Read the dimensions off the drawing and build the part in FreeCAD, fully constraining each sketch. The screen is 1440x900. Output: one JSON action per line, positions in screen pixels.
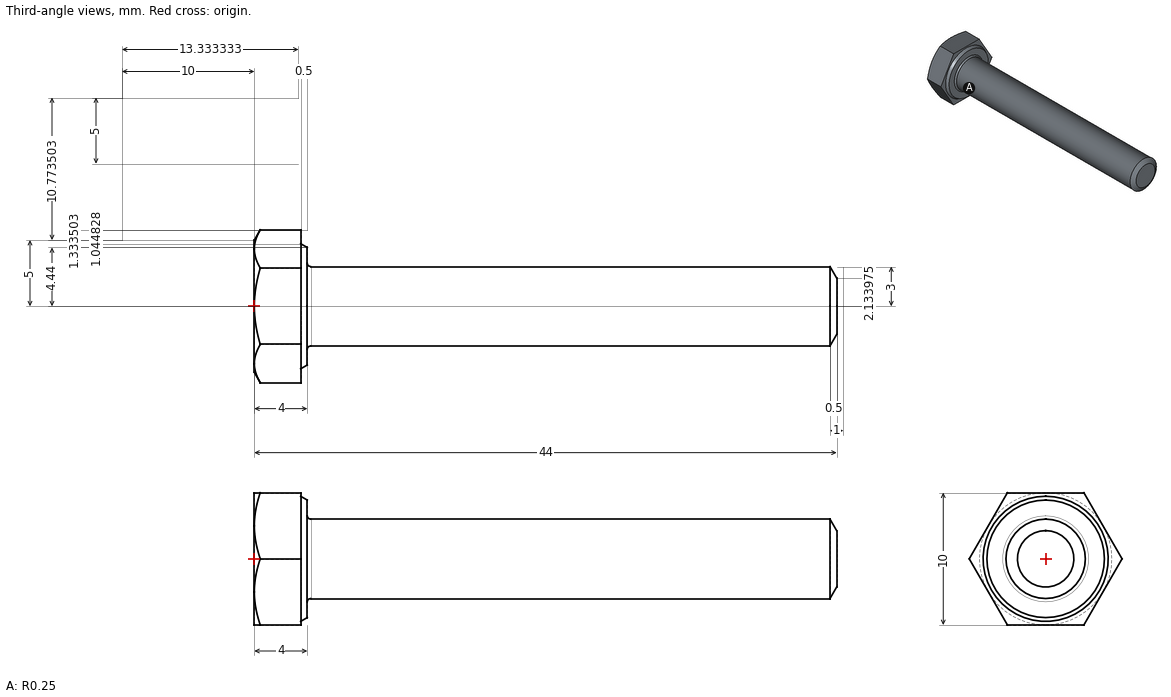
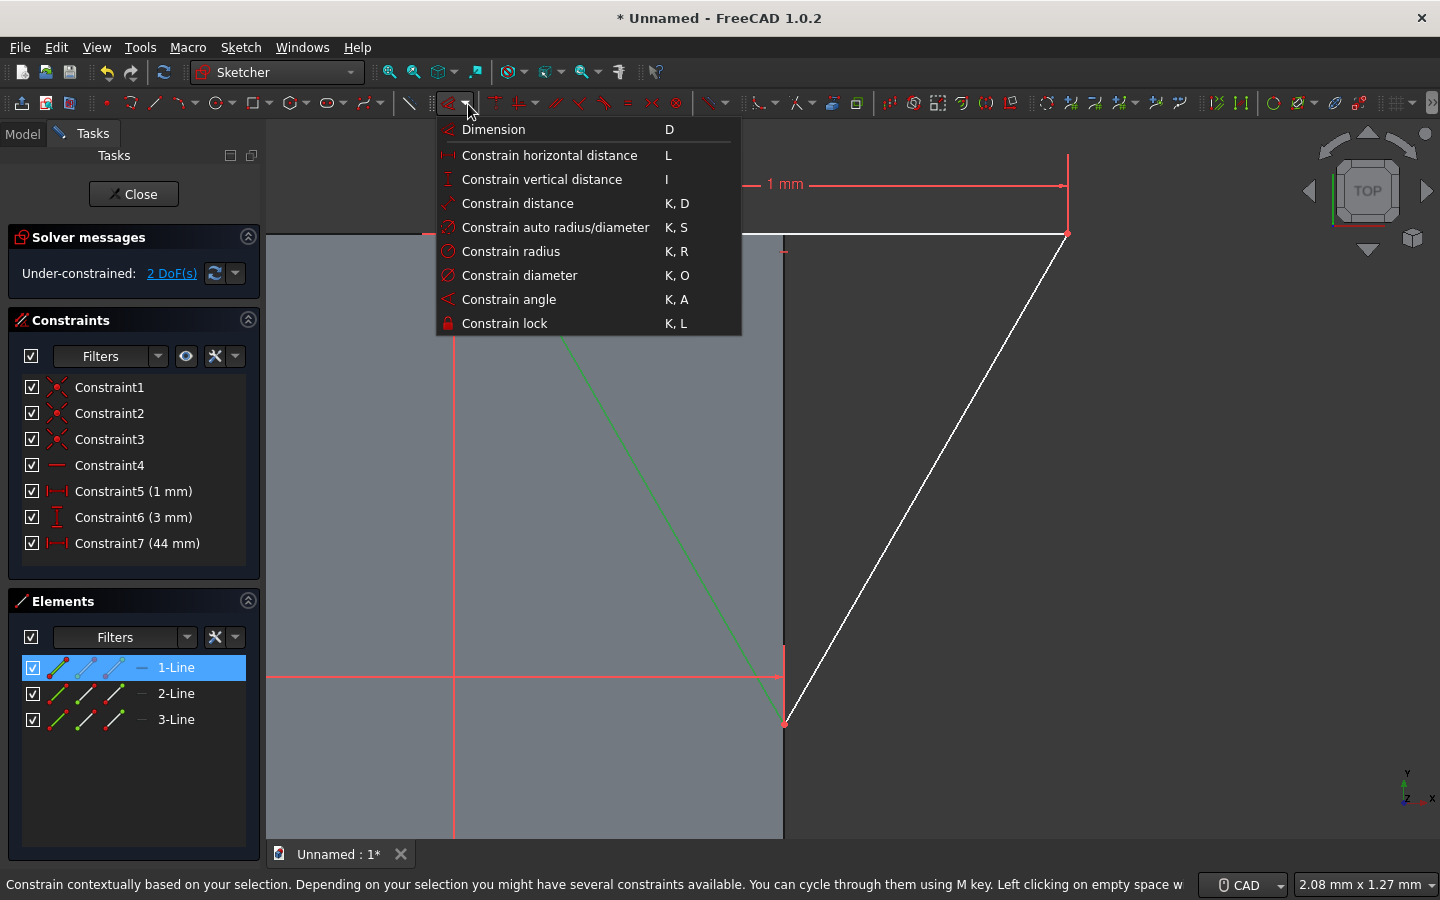
{"action": "left_click", "coordinate": [589, 155]}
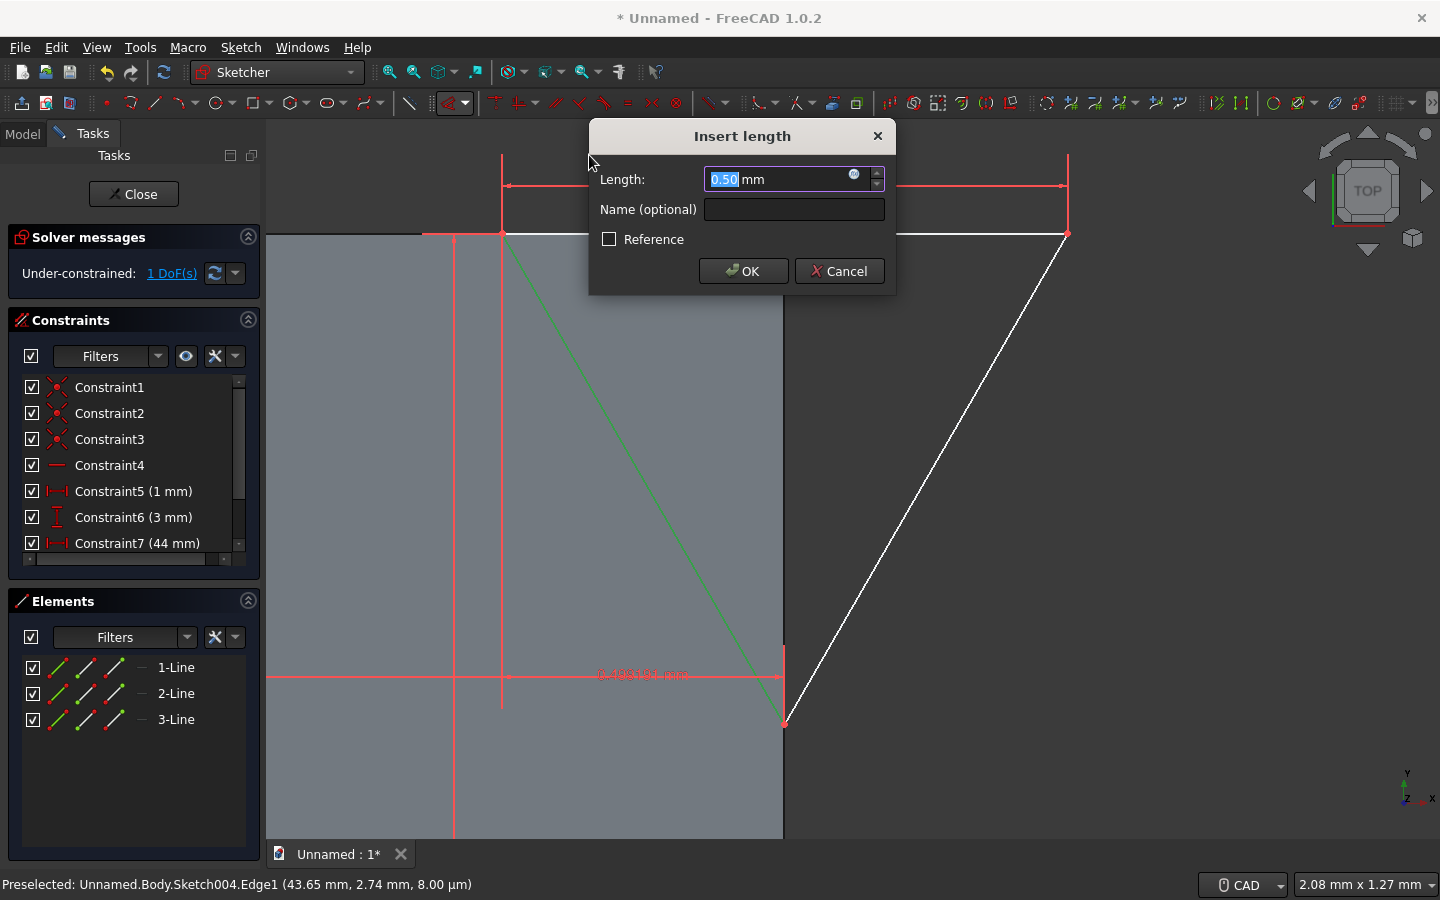
{"action": "type", "text": "0.5"}
{"action": "key", "text": "Return"}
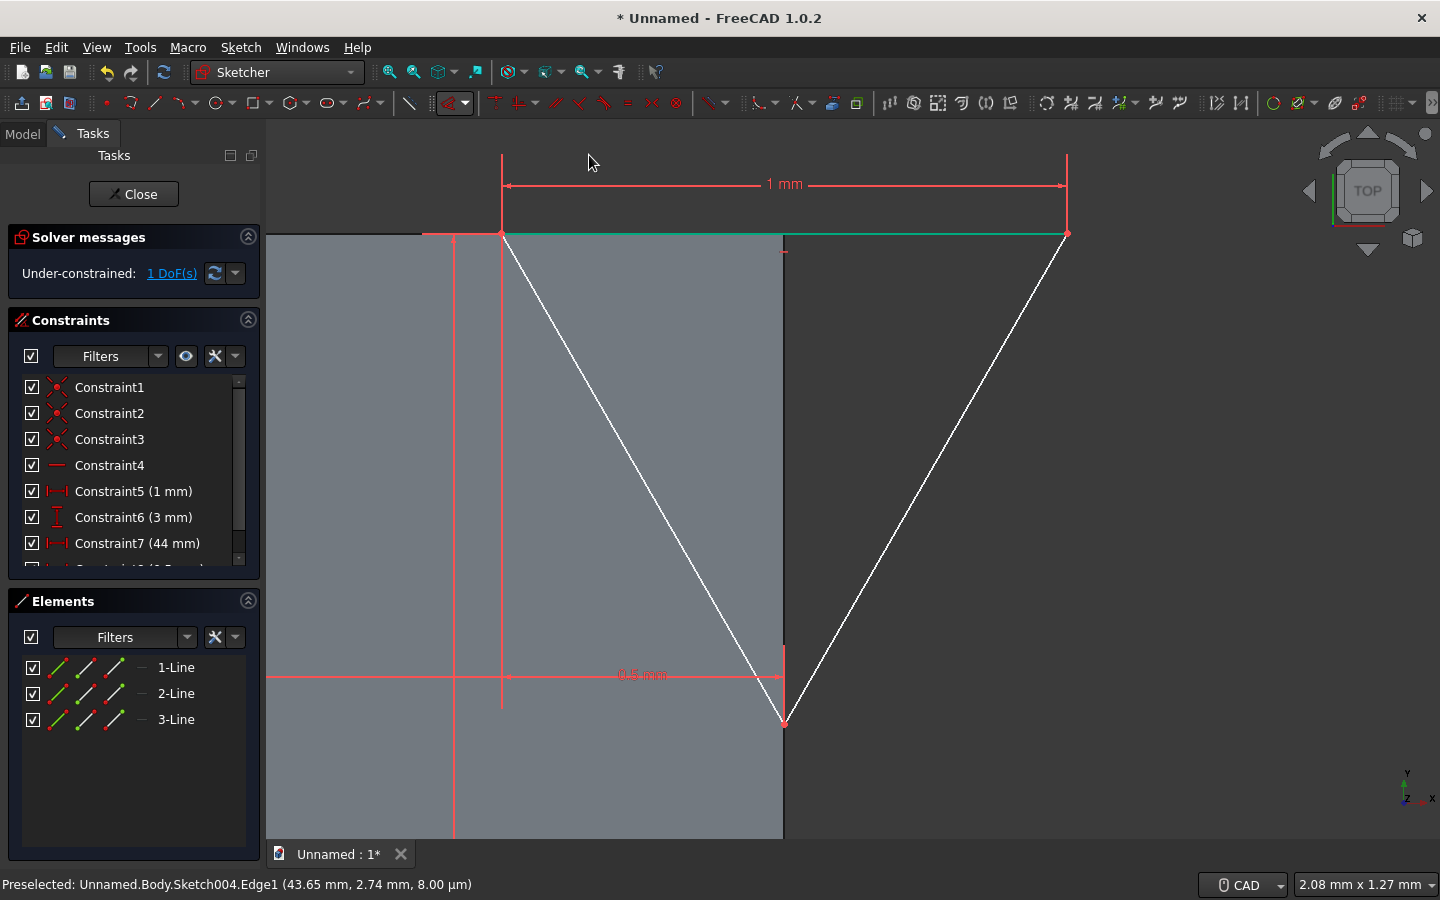
{"action": "left_click", "coordinate": [784, 725]}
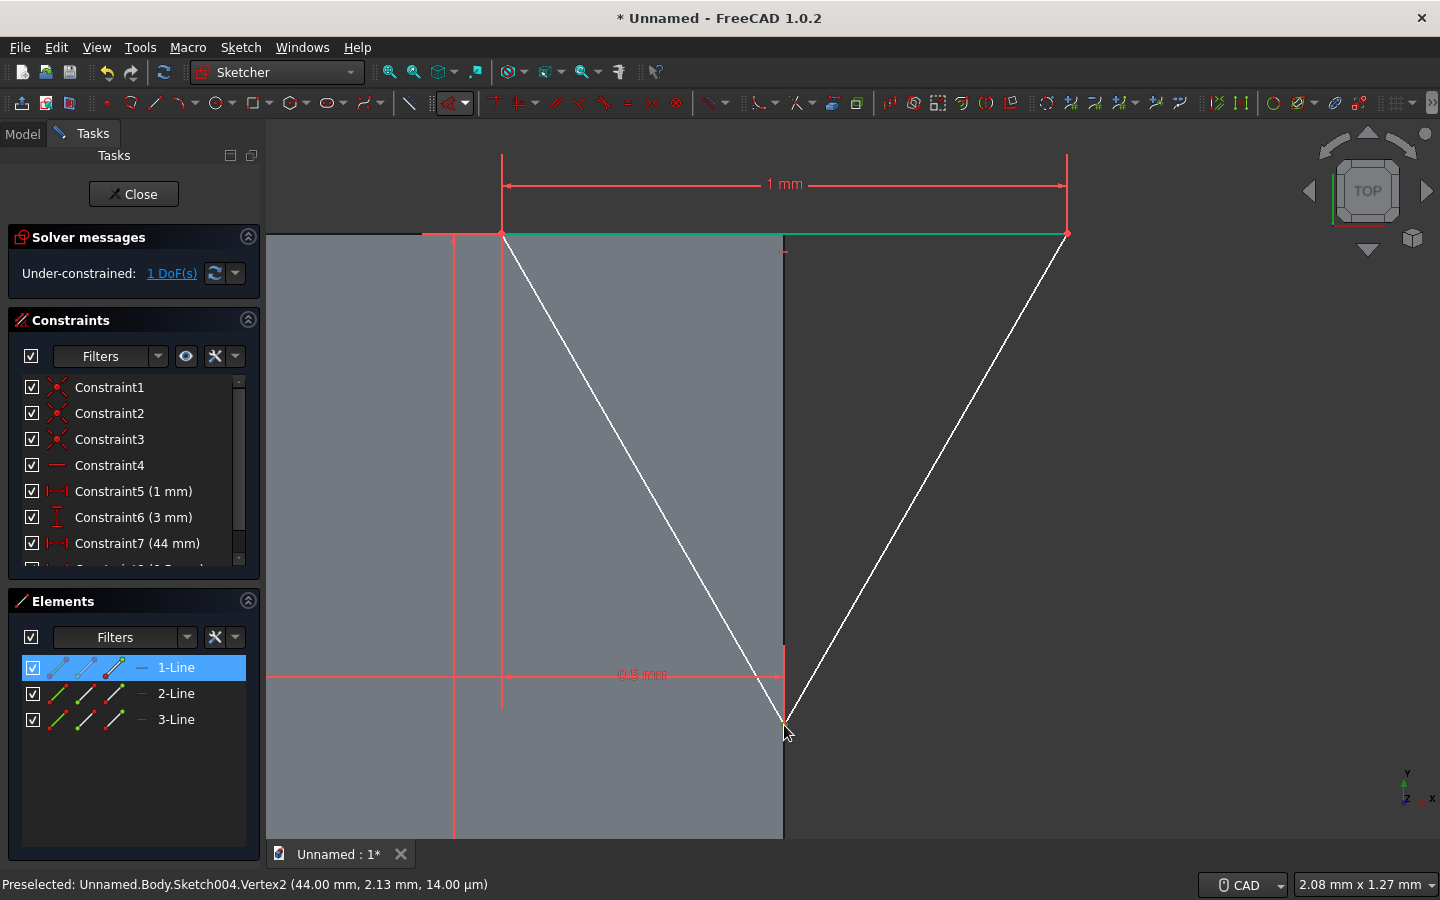
{"action": "left_click", "coordinate": [468, 104]}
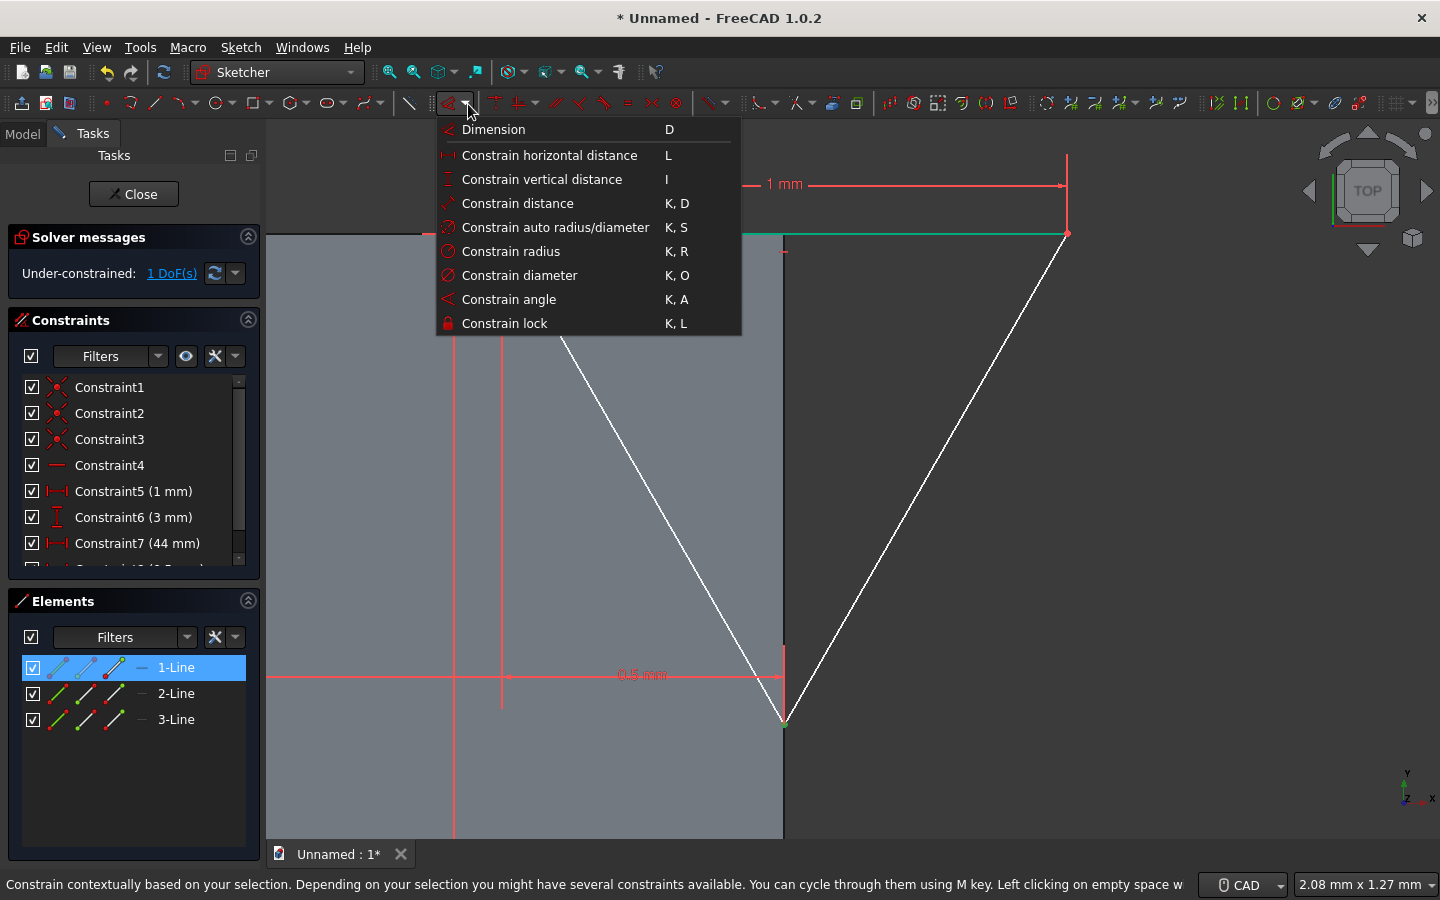
{"action": "left_click", "coordinate": [589, 179]}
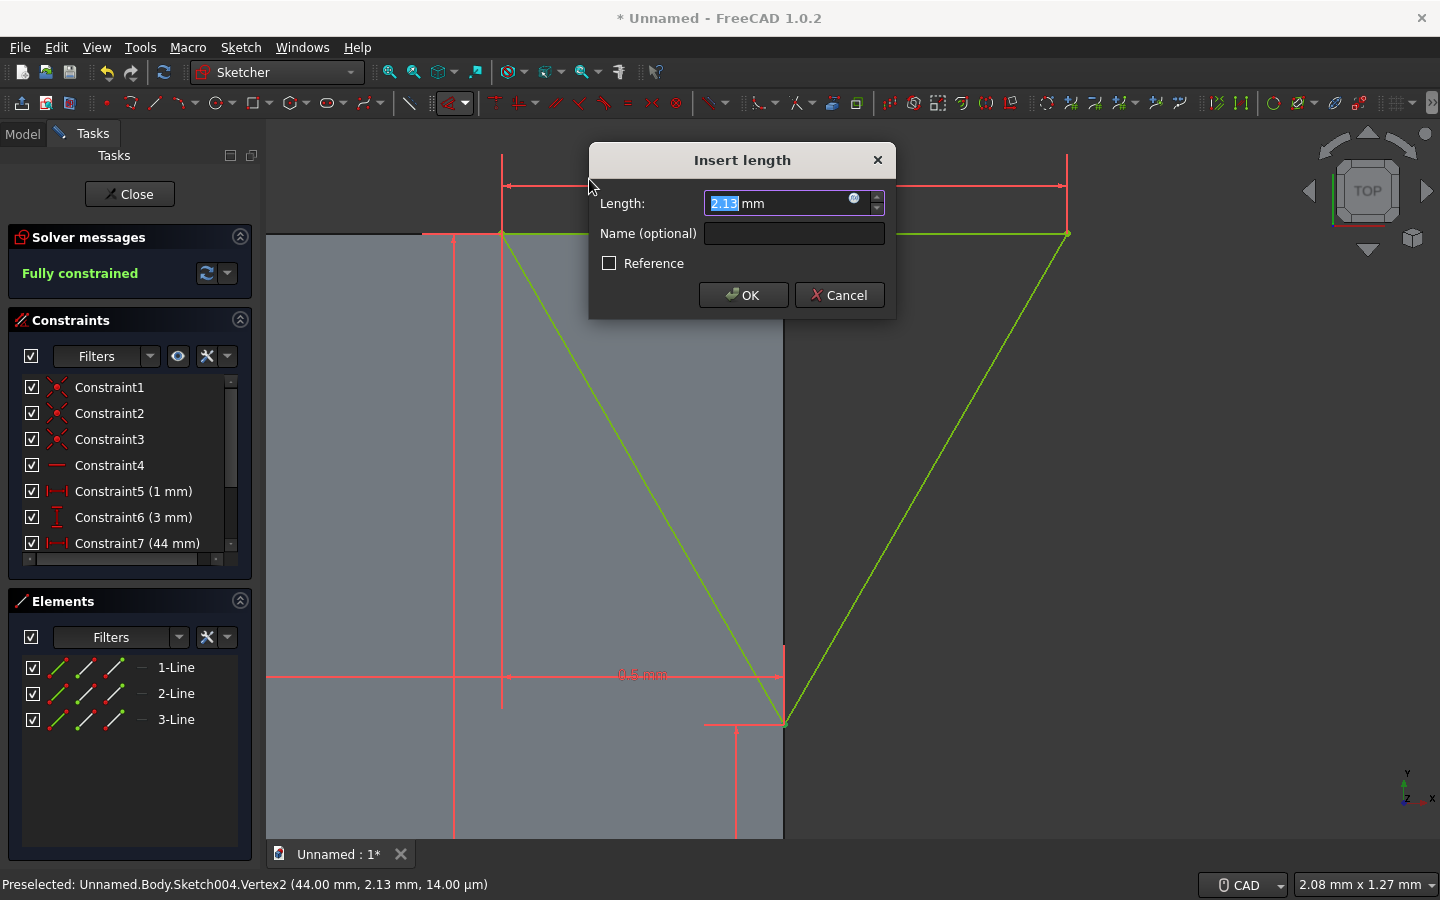
{"action": "type", "text": "2.133975"}
{"action": "key", "text": "Return"}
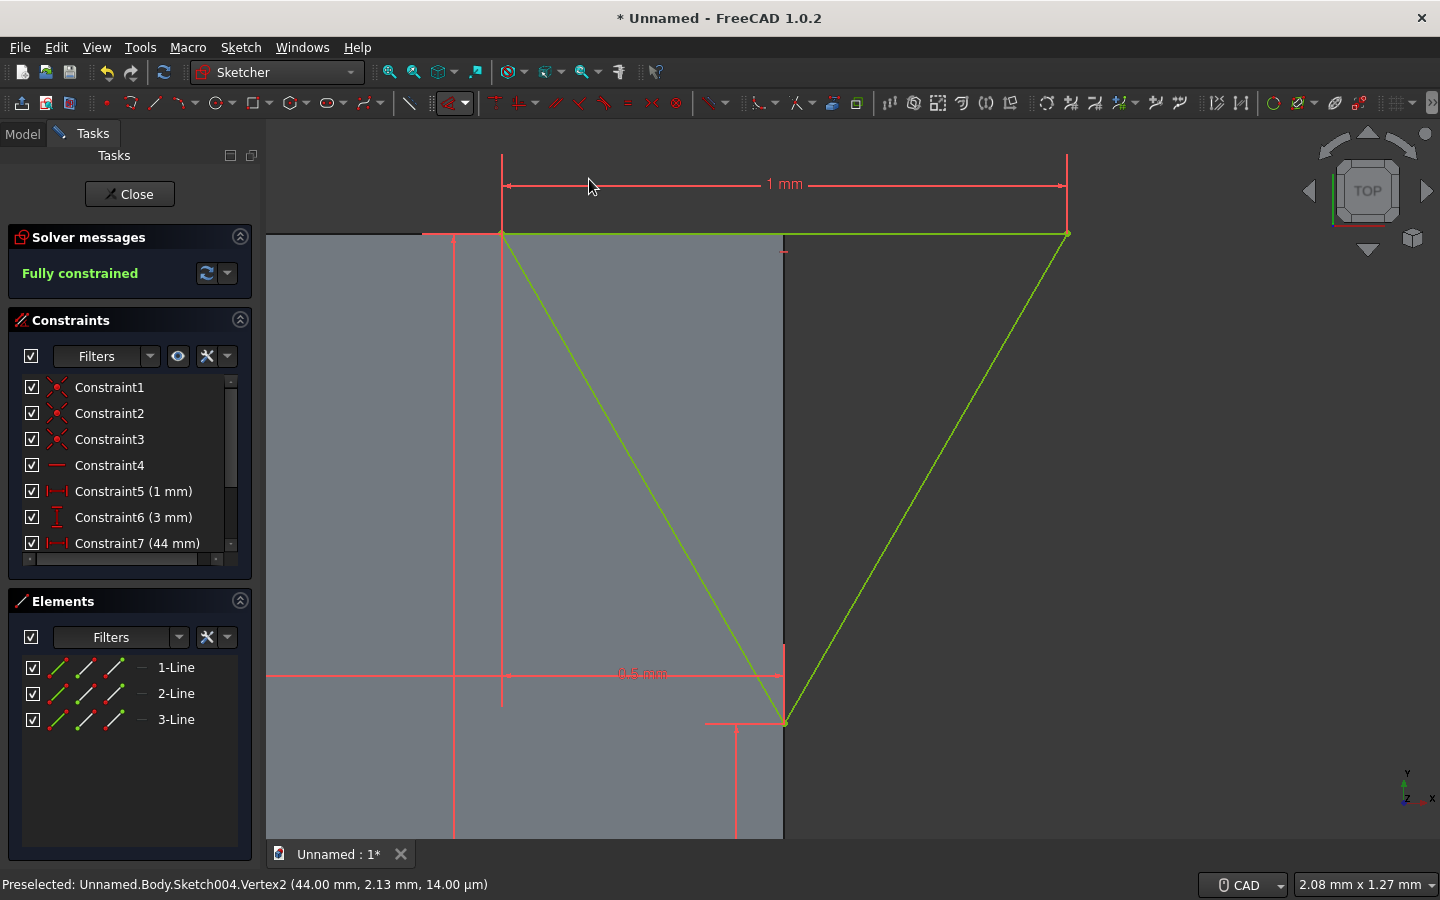
{"action": "left_click", "coordinate": [130, 194]}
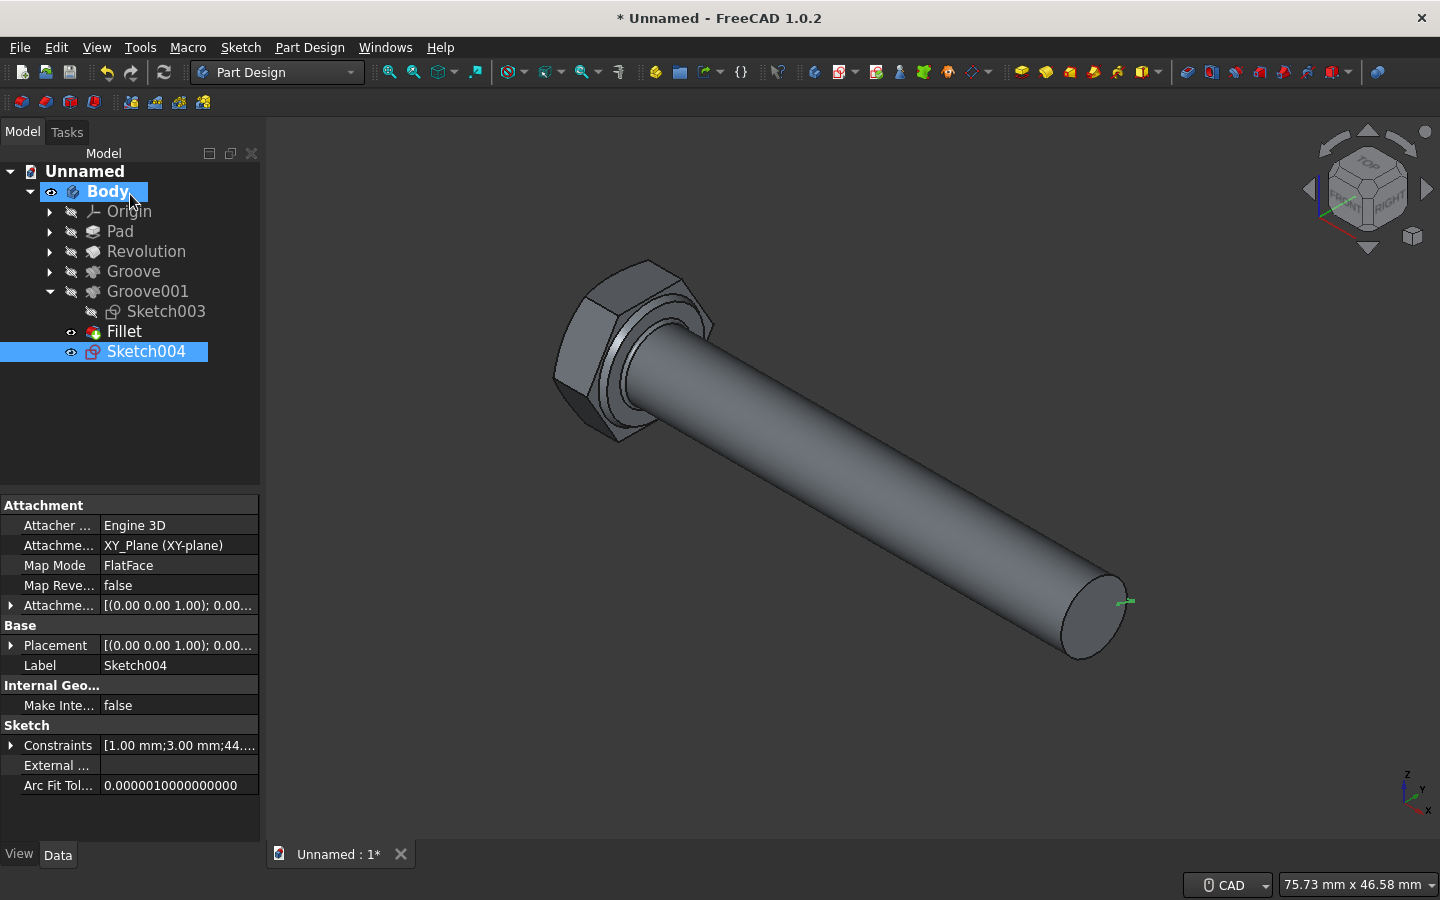
{"action": "left_click", "coordinate": [1236, 72]}